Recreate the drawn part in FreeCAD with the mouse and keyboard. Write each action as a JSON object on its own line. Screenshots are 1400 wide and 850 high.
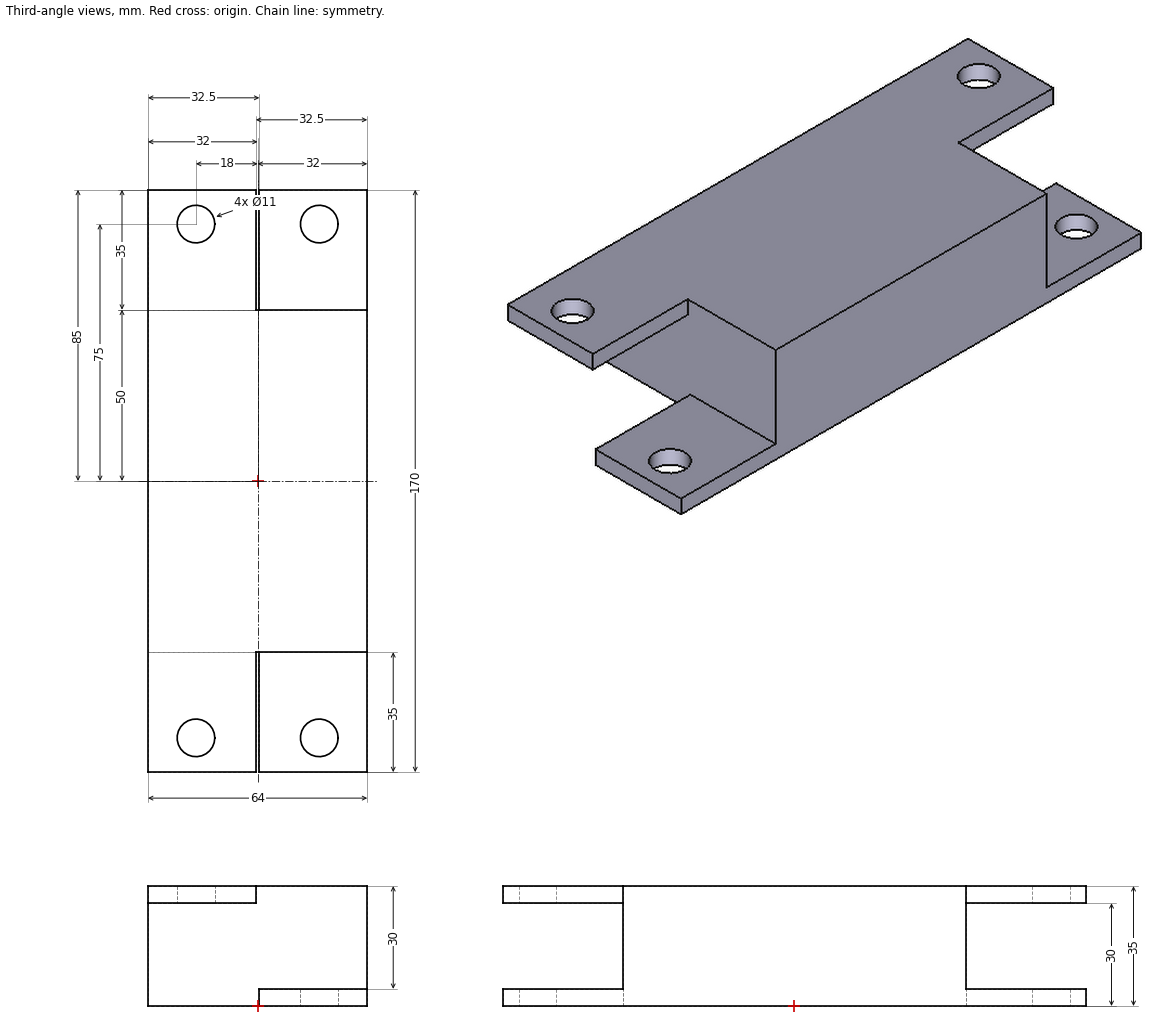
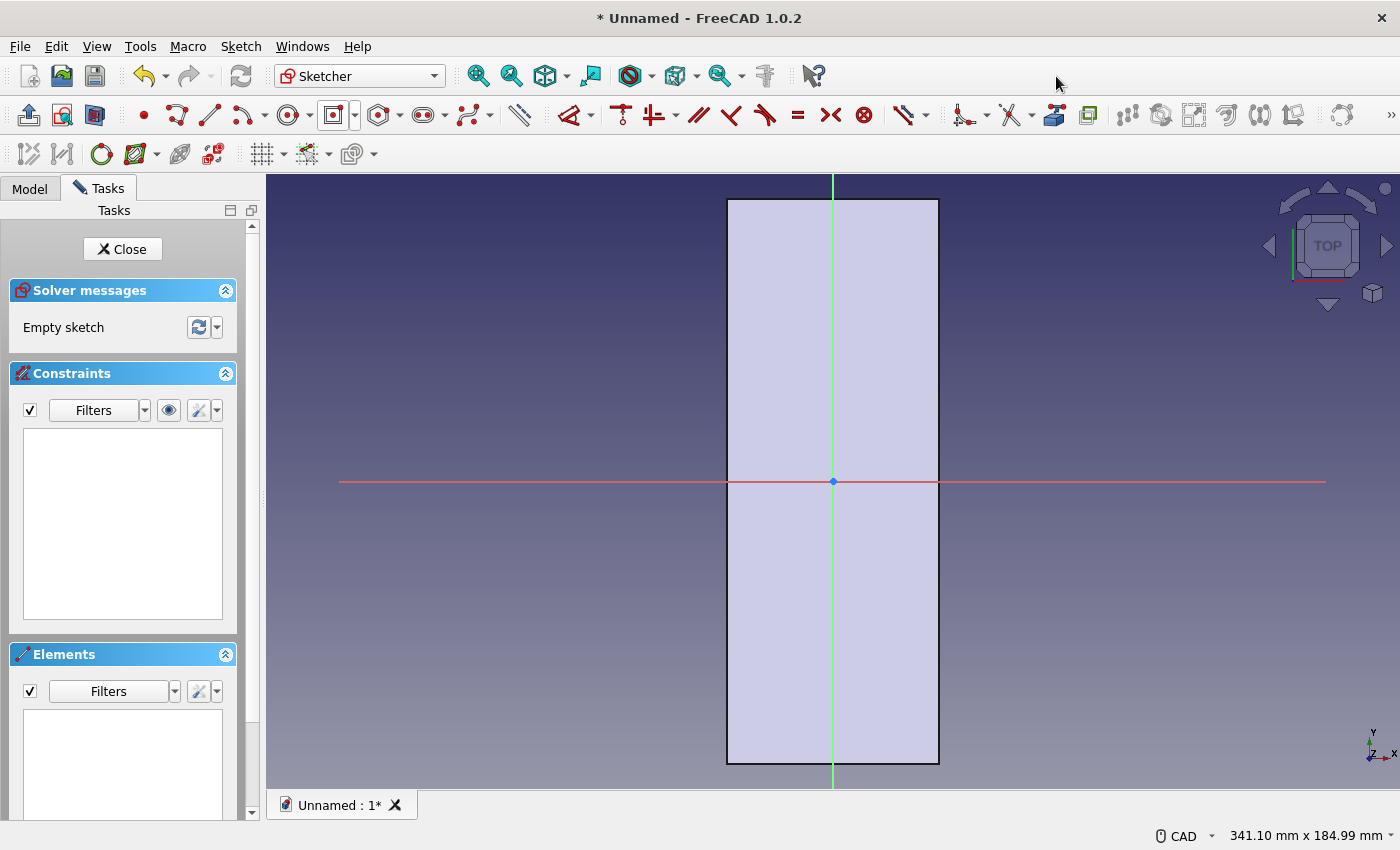
{"action": "scroll", "coordinate": [519, 481], "scroll_direction": "down", "scroll_amount": 2}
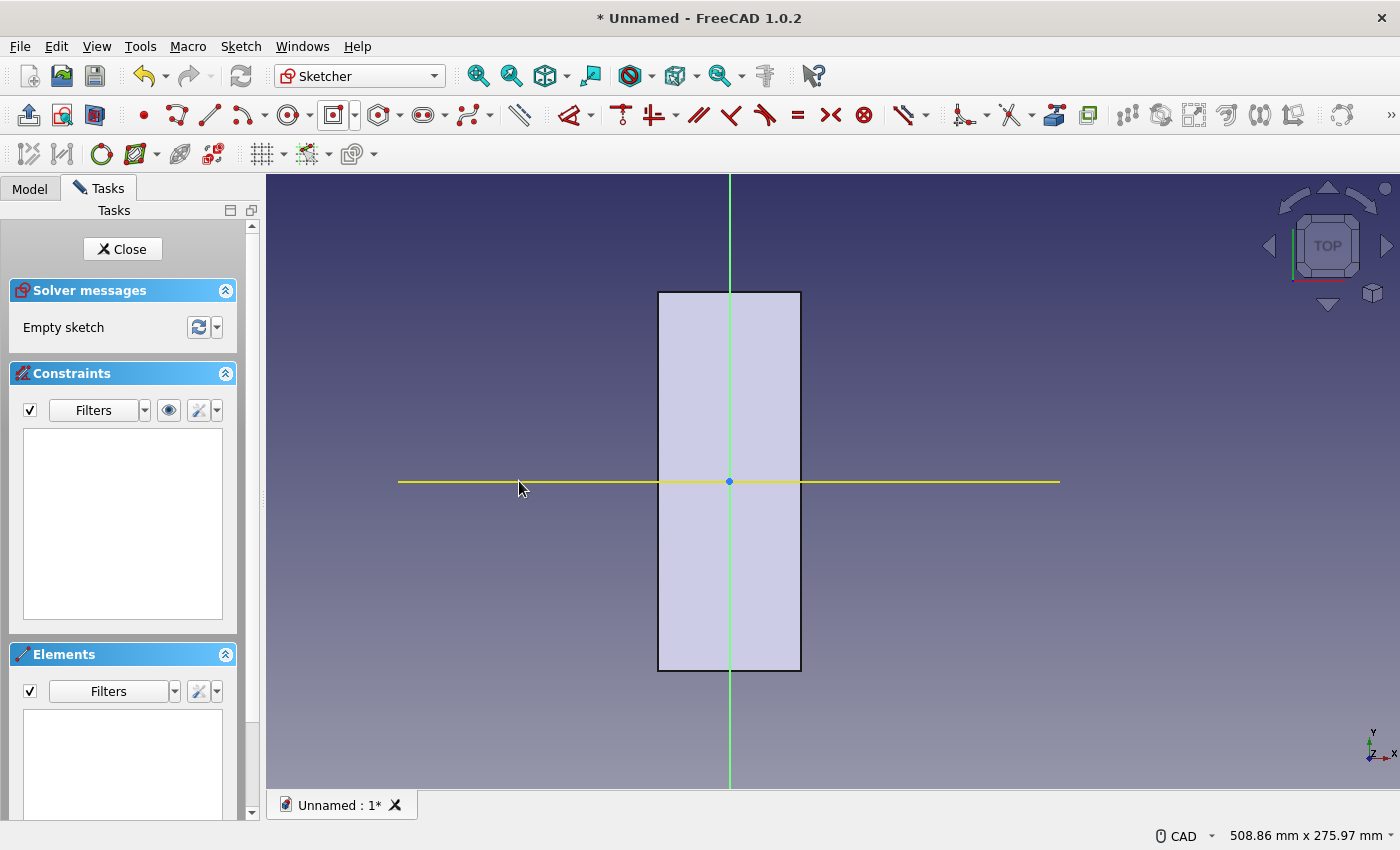
{"action": "left_click", "coordinate": [354, 116]}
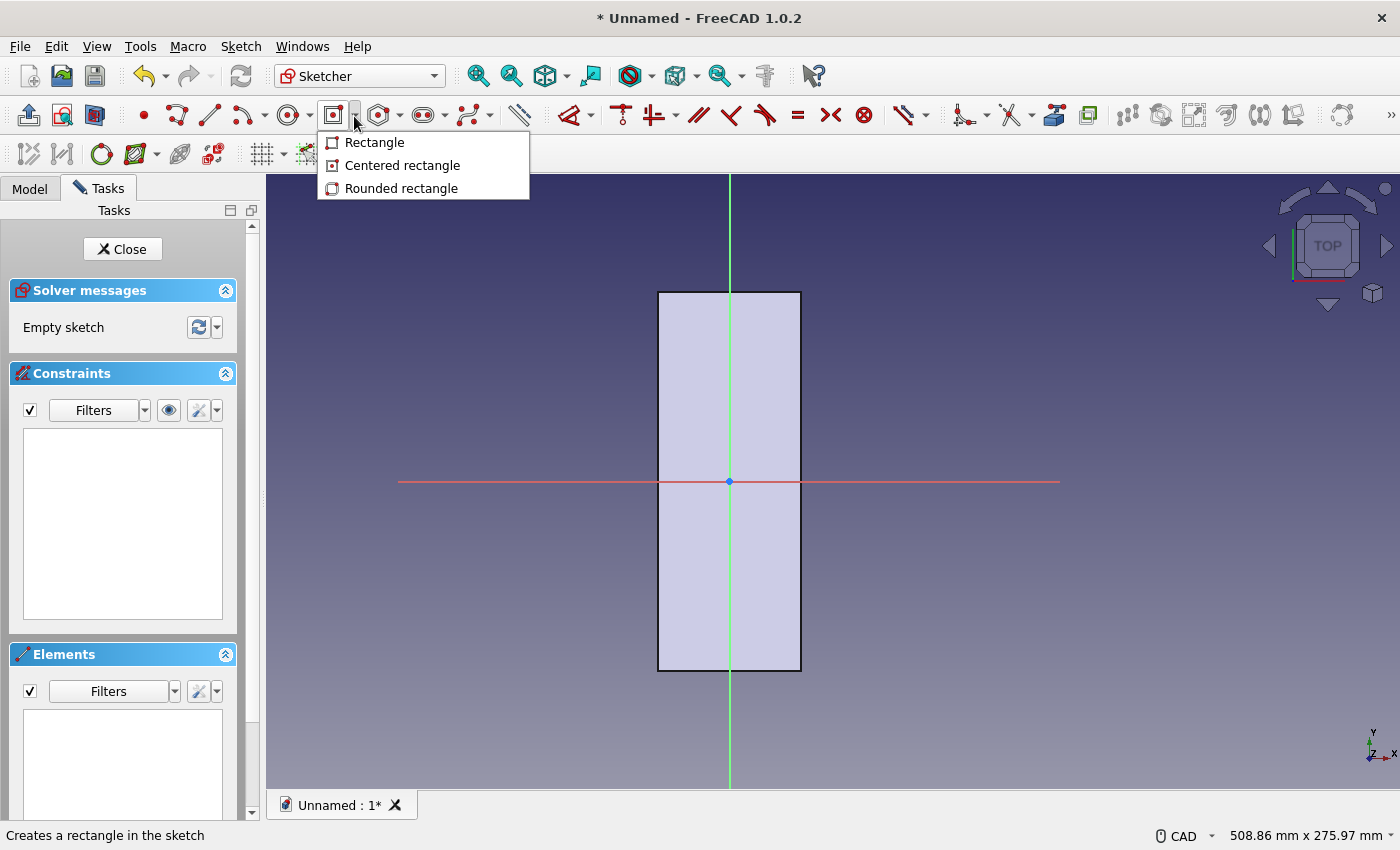
{"action": "left_click", "coordinate": [424, 142]}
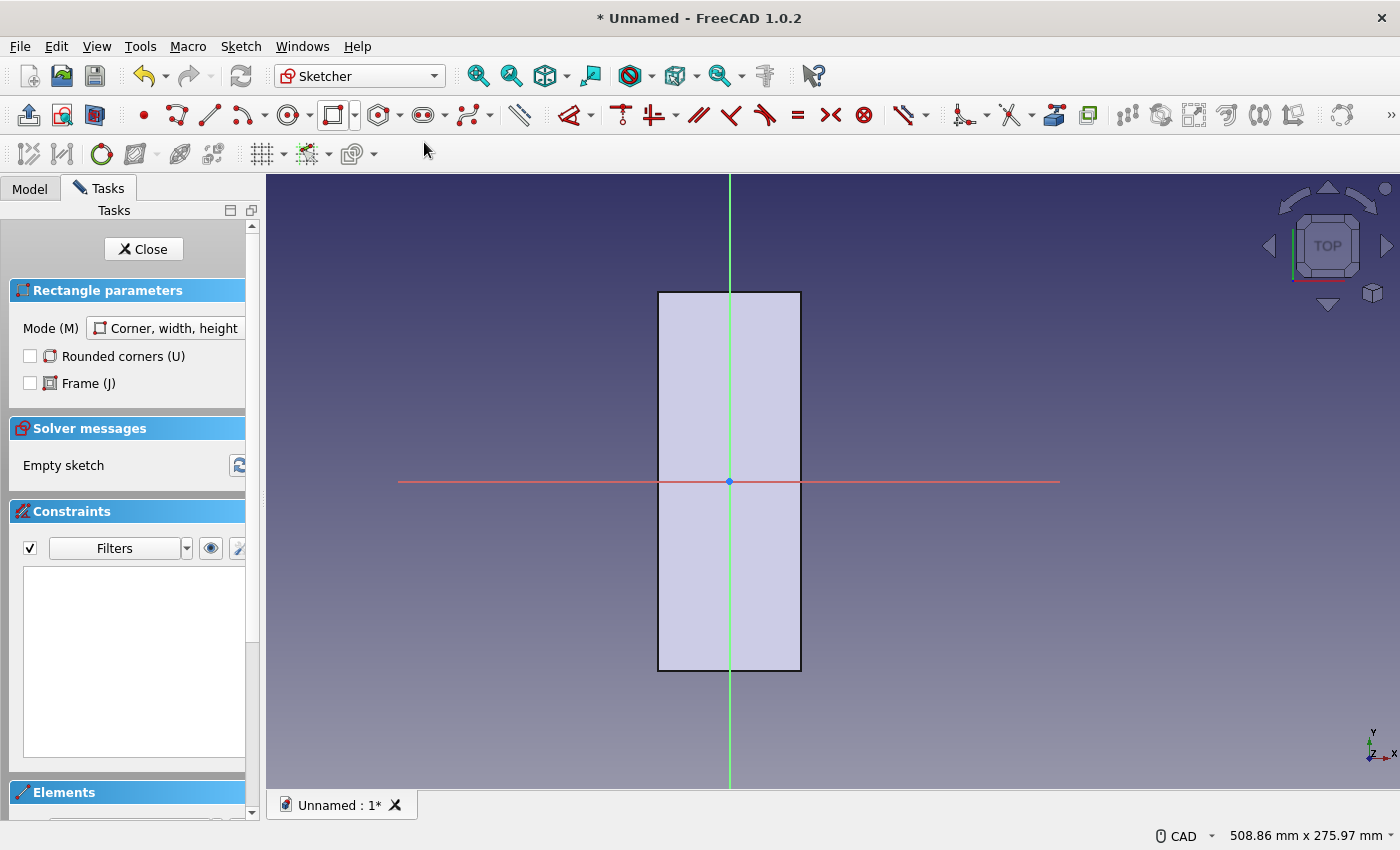
{"action": "scroll", "coordinate": [728, 292], "scroll_direction": "up", "scroll_amount": 14}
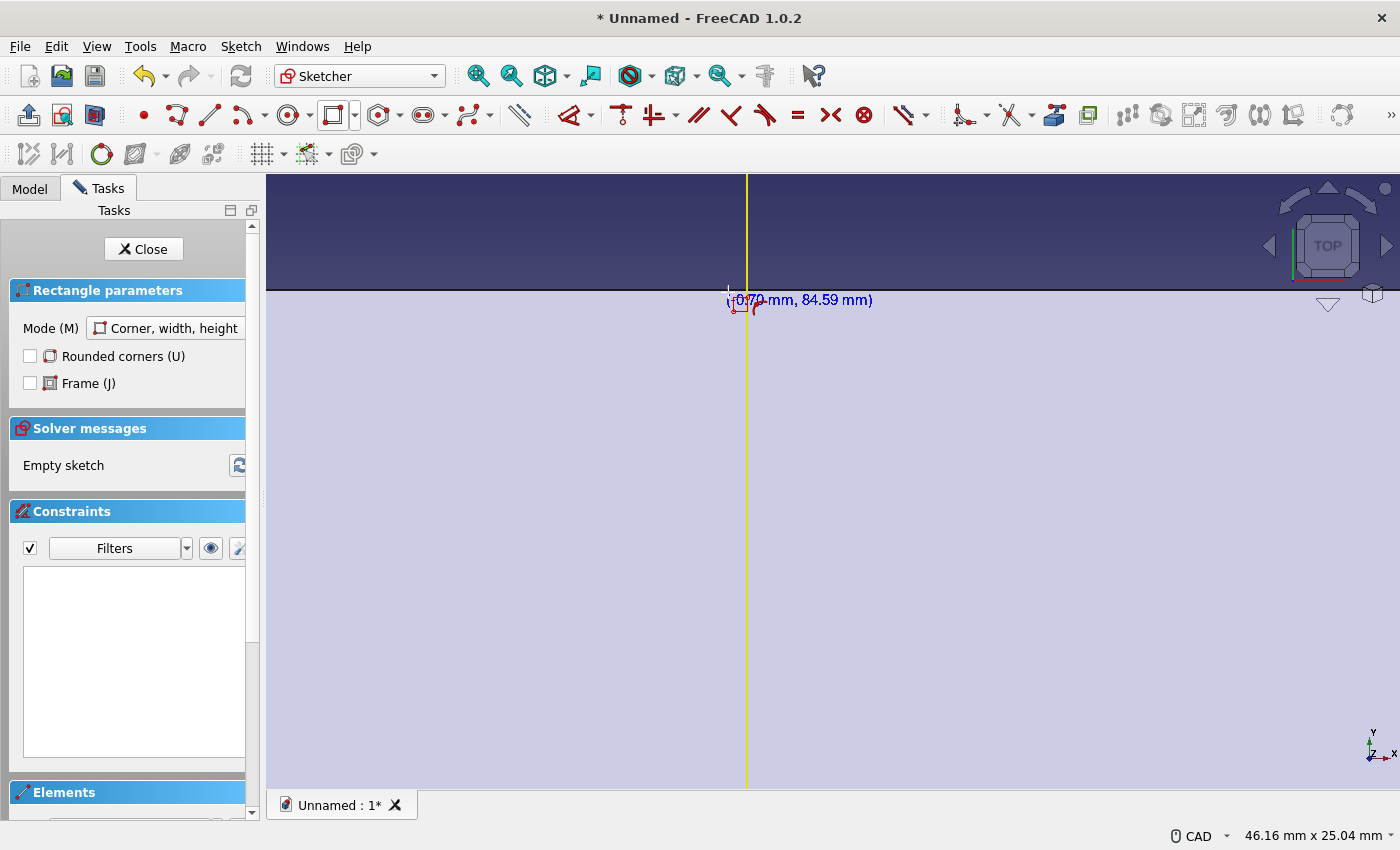
{"action": "left_click", "coordinate": [729, 290]}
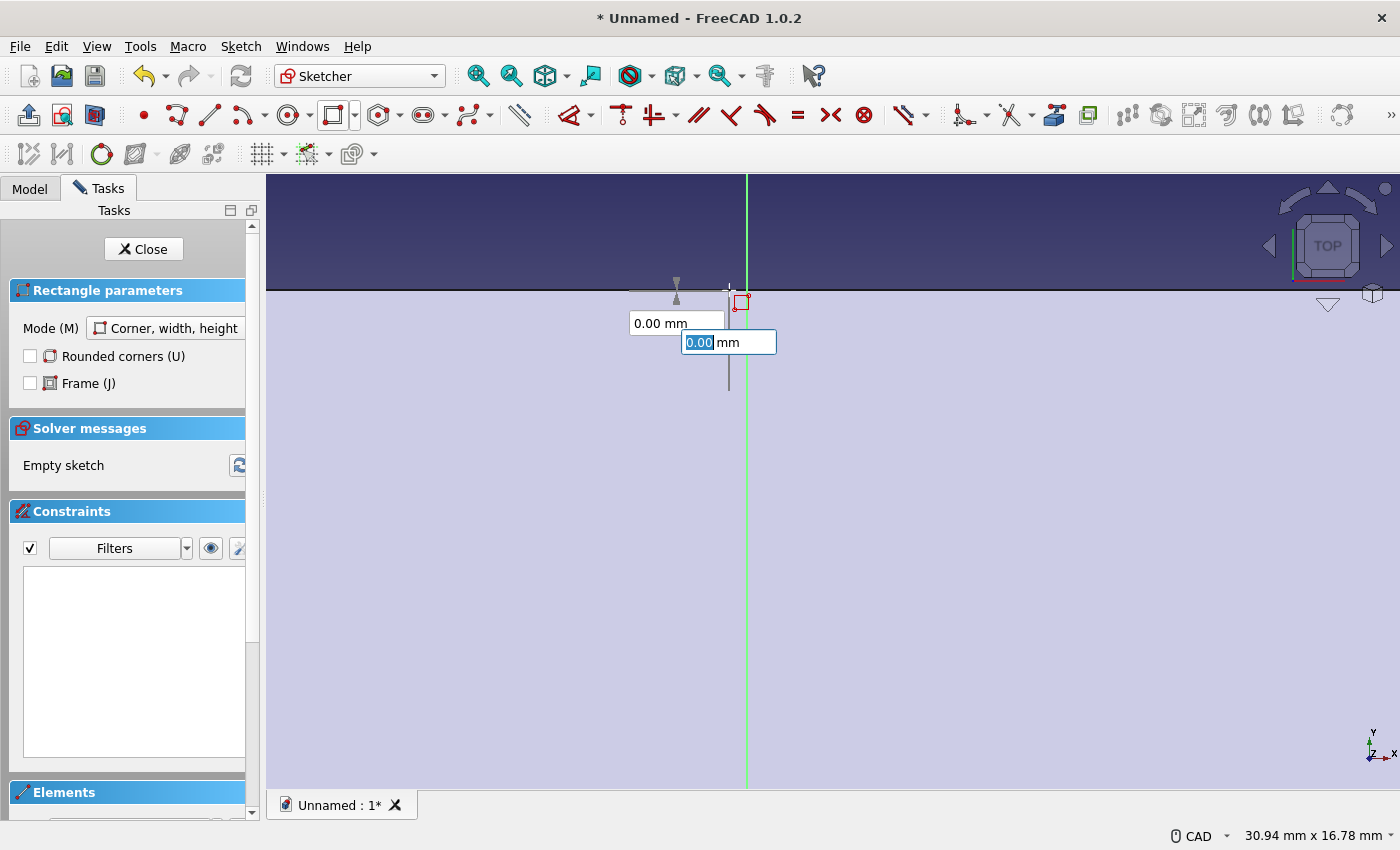
{"action": "scroll", "coordinate": [728, 292], "scroll_direction": "down", "scroll_amount": 14}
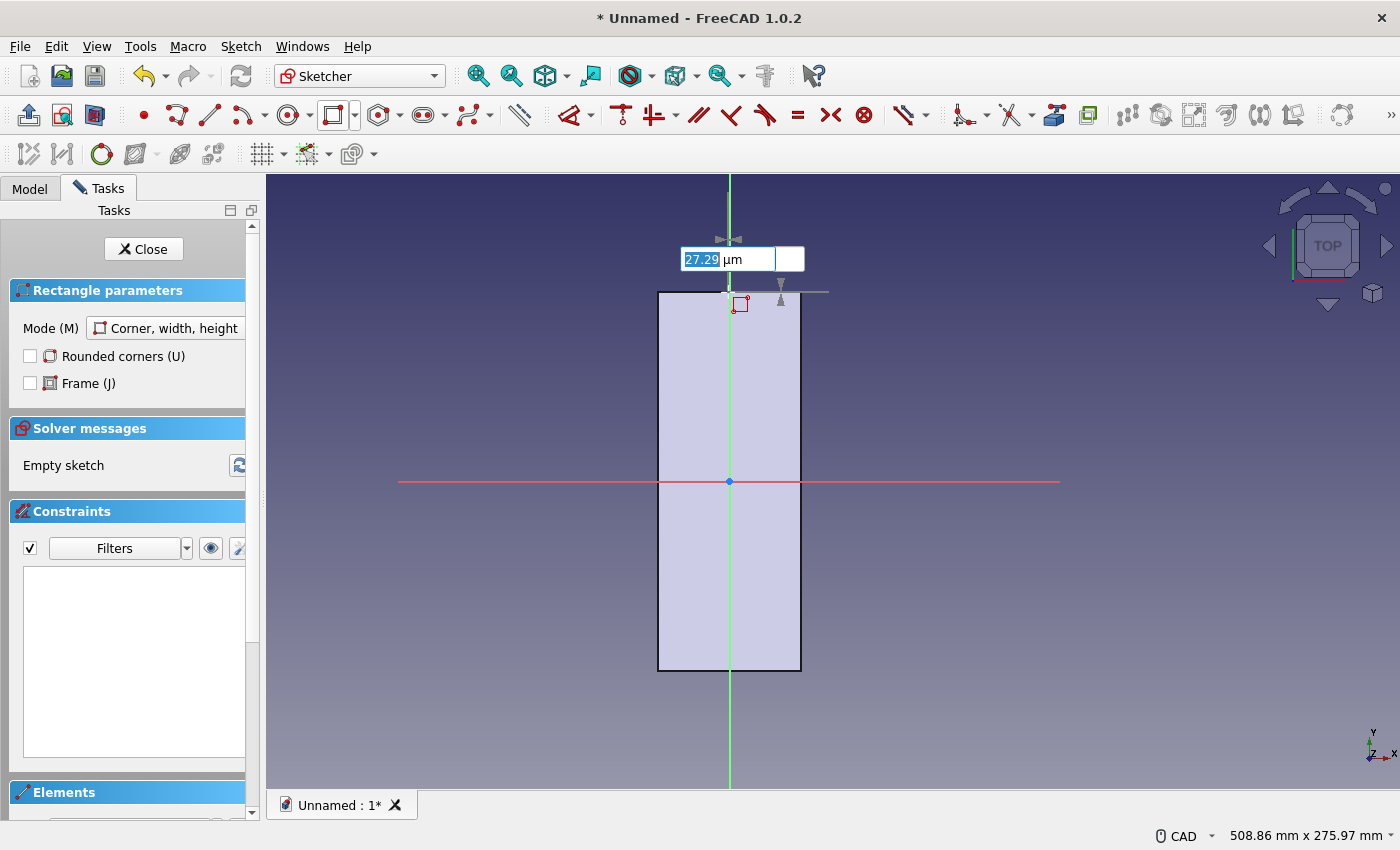
{"action": "left_click", "coordinate": [801, 370]}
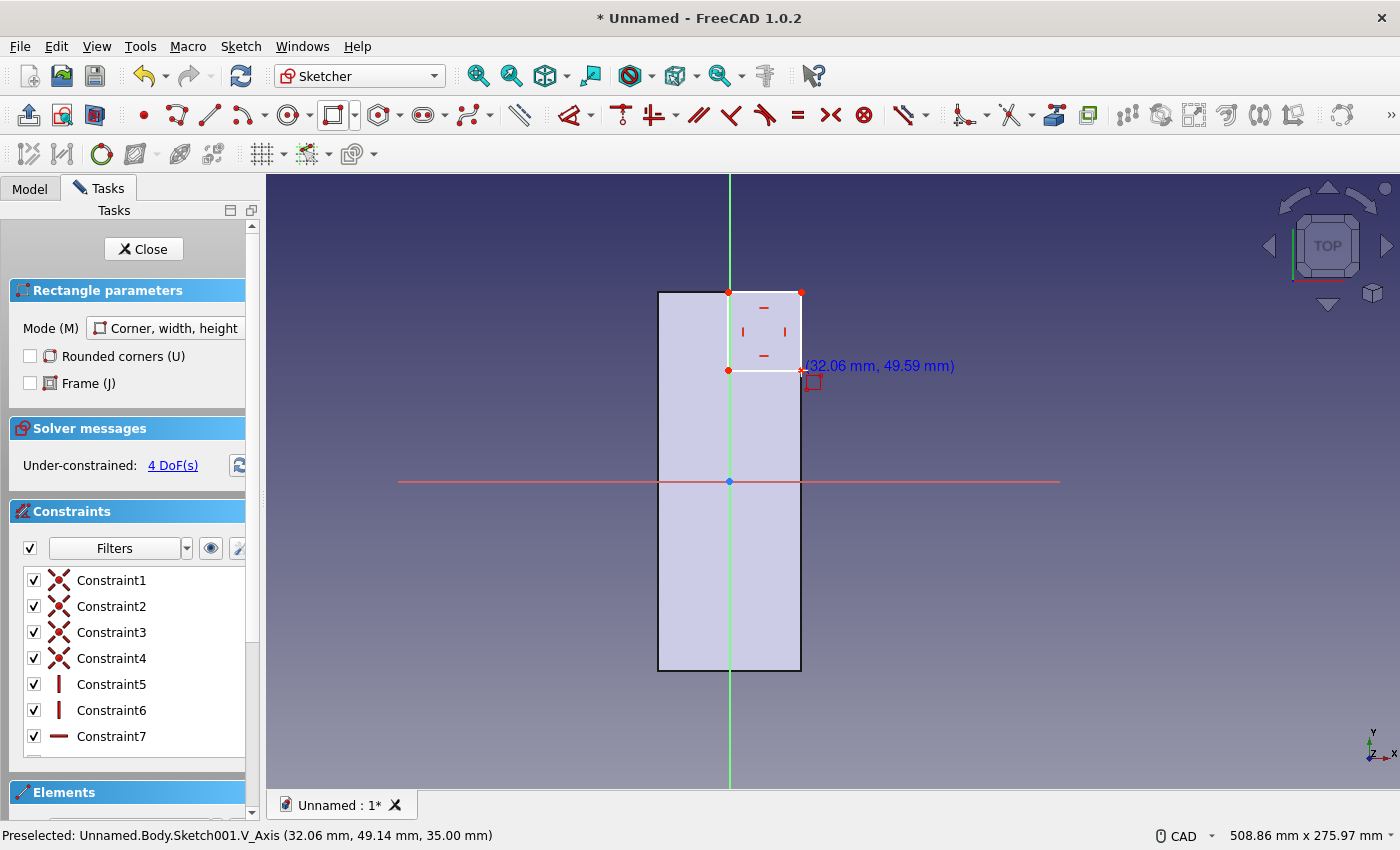
{"action": "scroll", "coordinate": [728, 593], "scroll_direction": "up", "scroll_amount": 14}